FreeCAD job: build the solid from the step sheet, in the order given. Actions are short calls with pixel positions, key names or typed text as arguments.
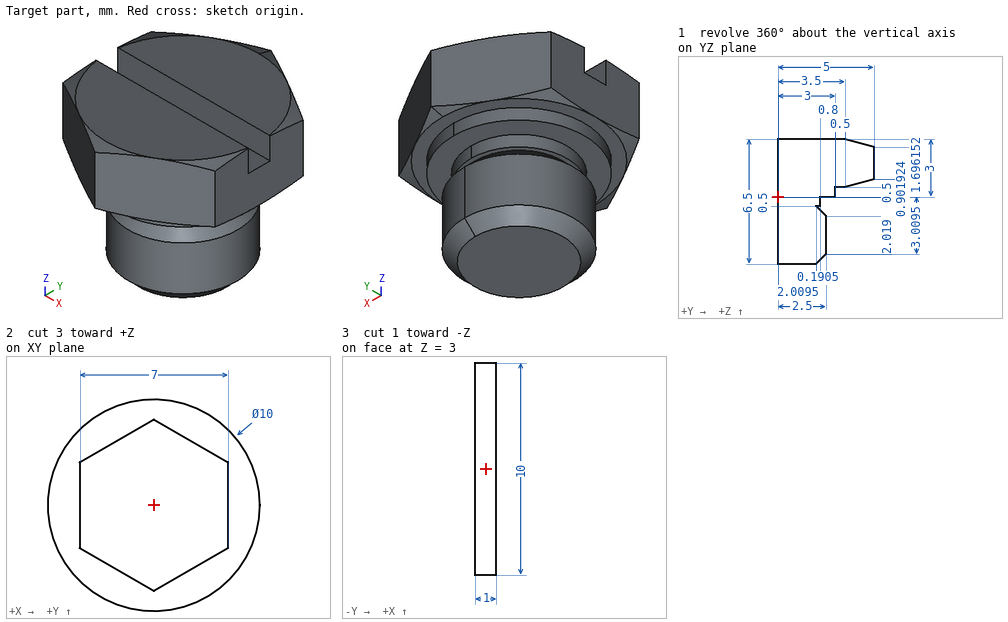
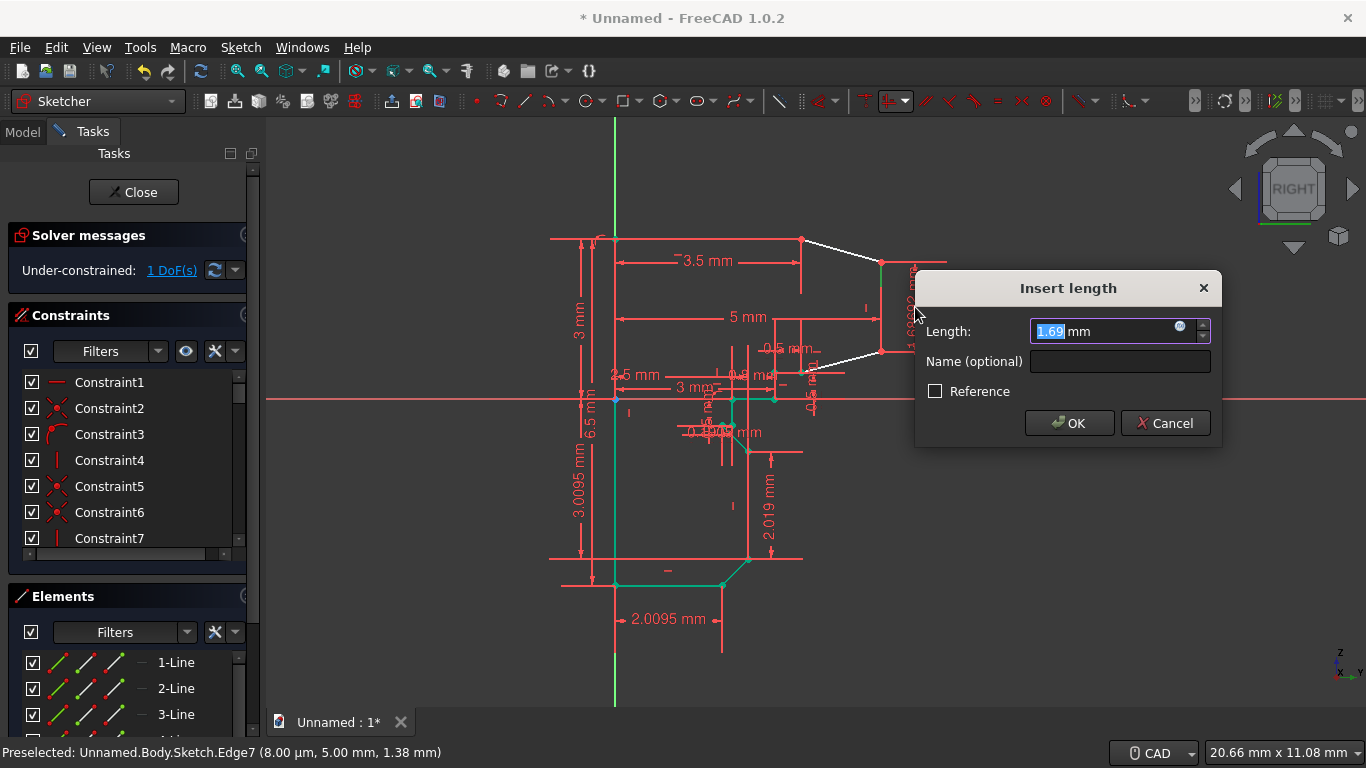
text(1.696152)
key(Return)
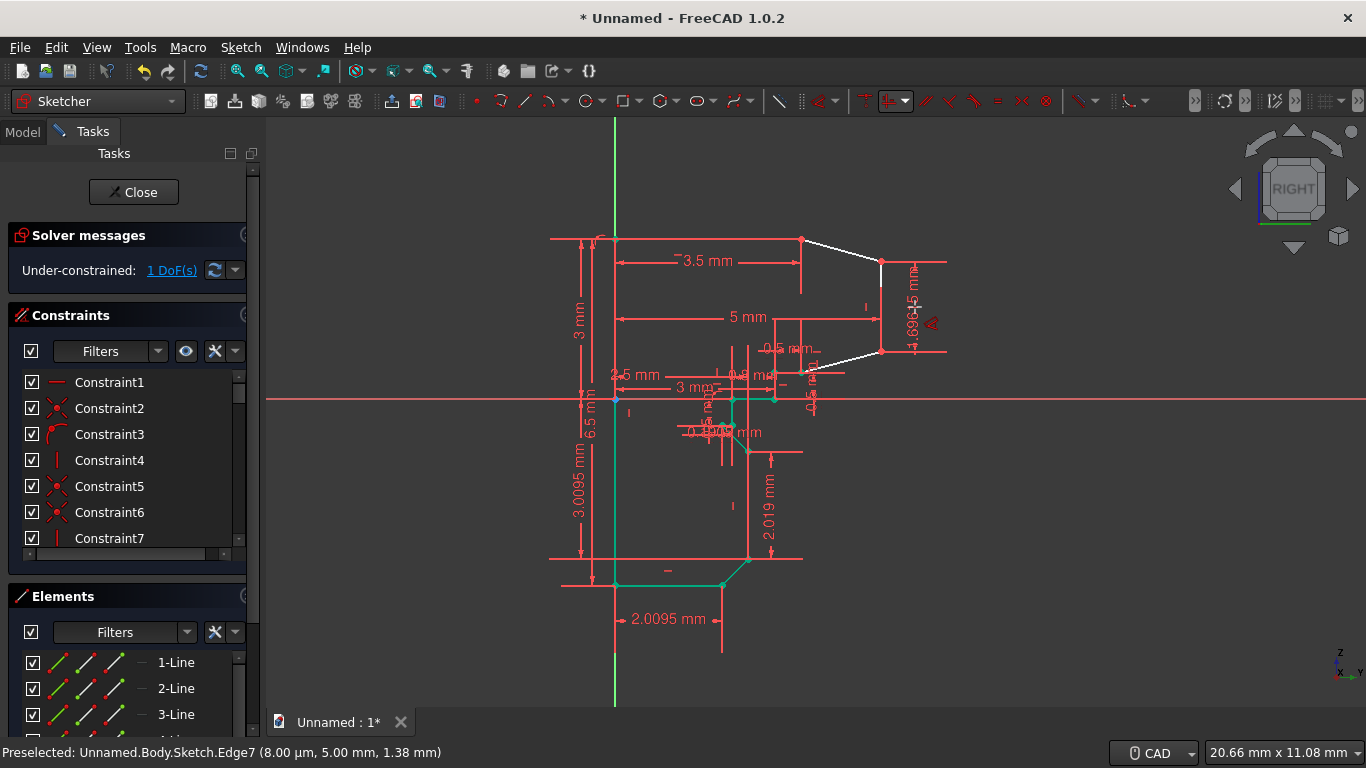
click(881, 352)
click(915, 376)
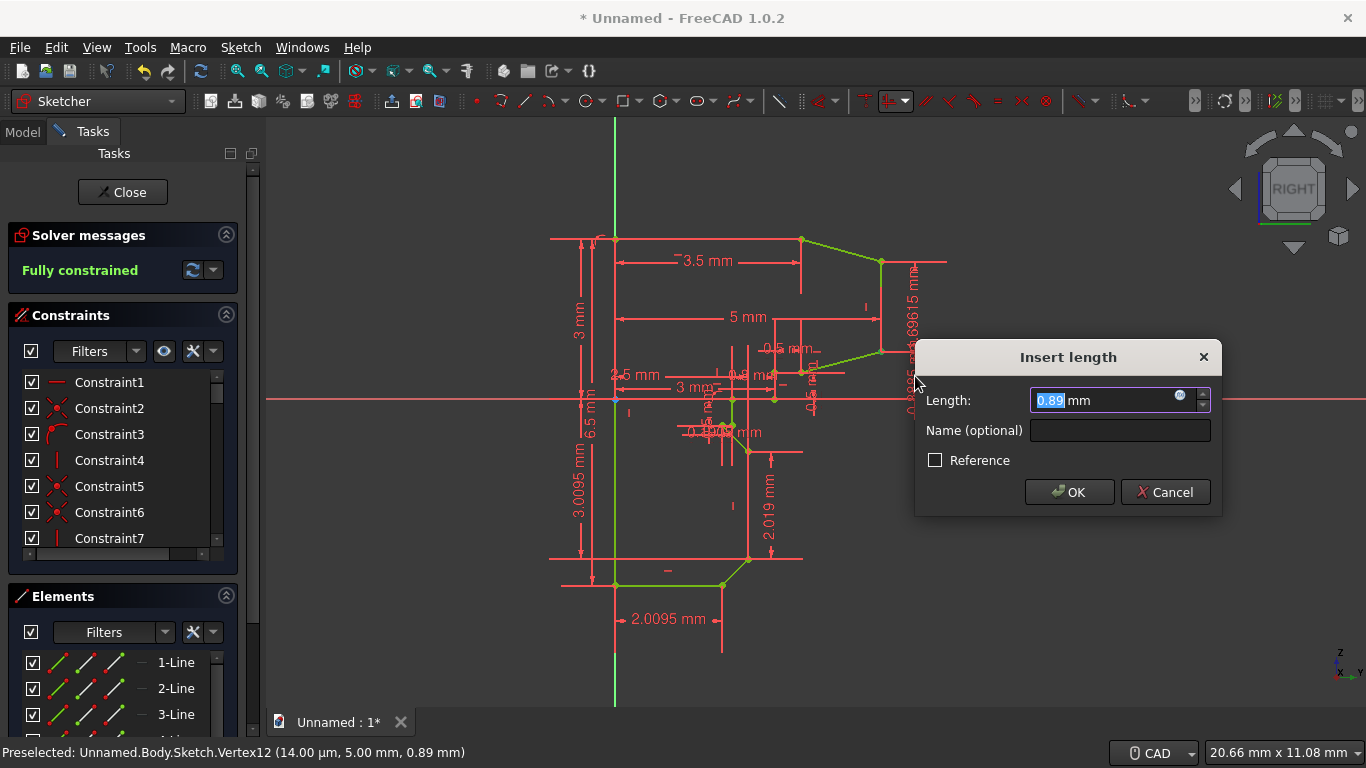
text(0.901924)
key(Return)
key(Escape)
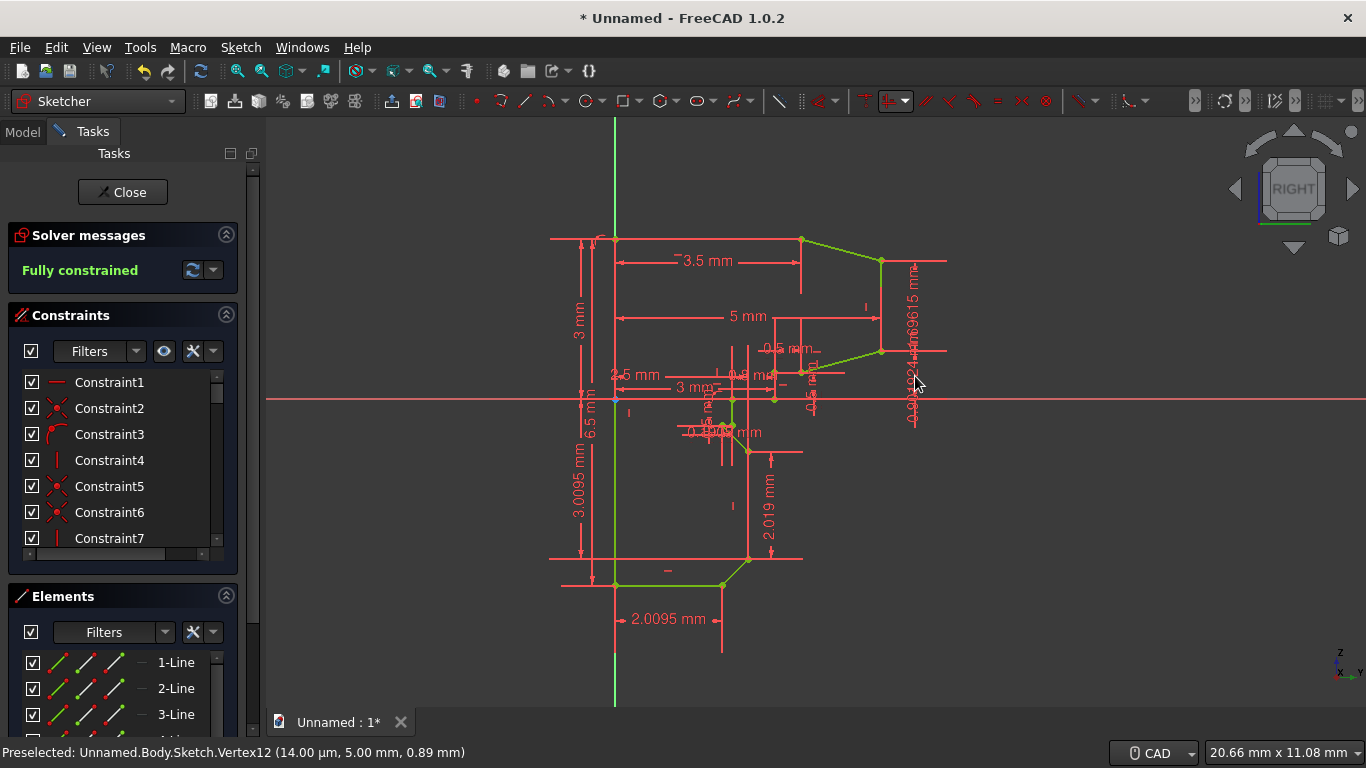
click(123, 192)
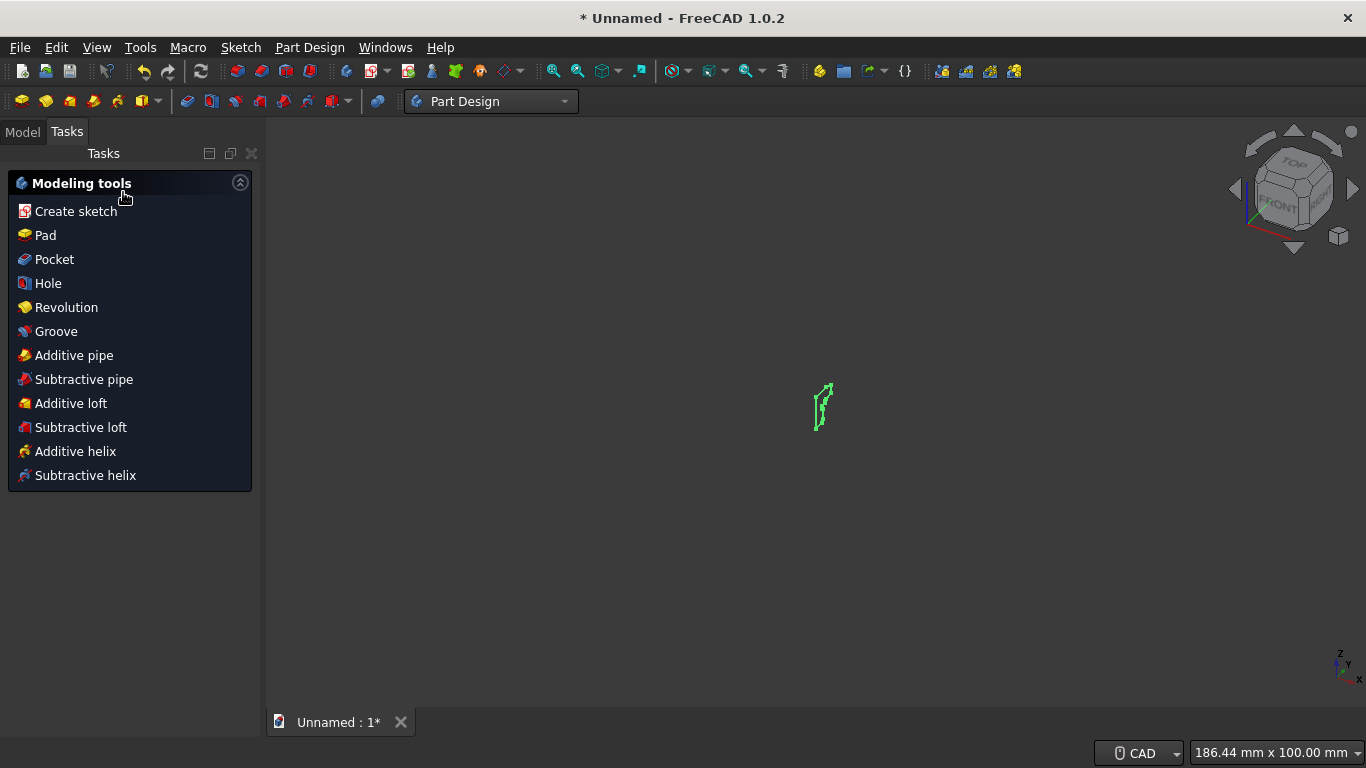
click(46, 102)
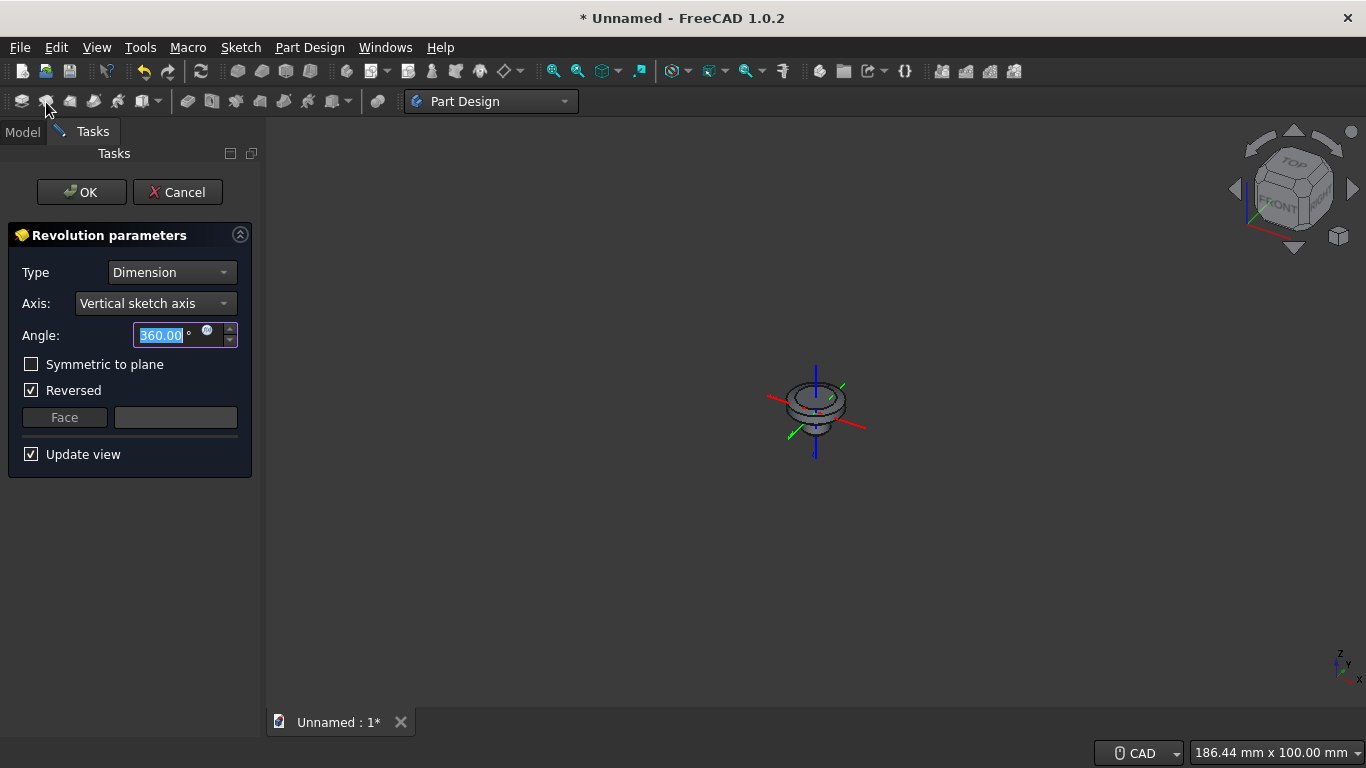
click(82, 192)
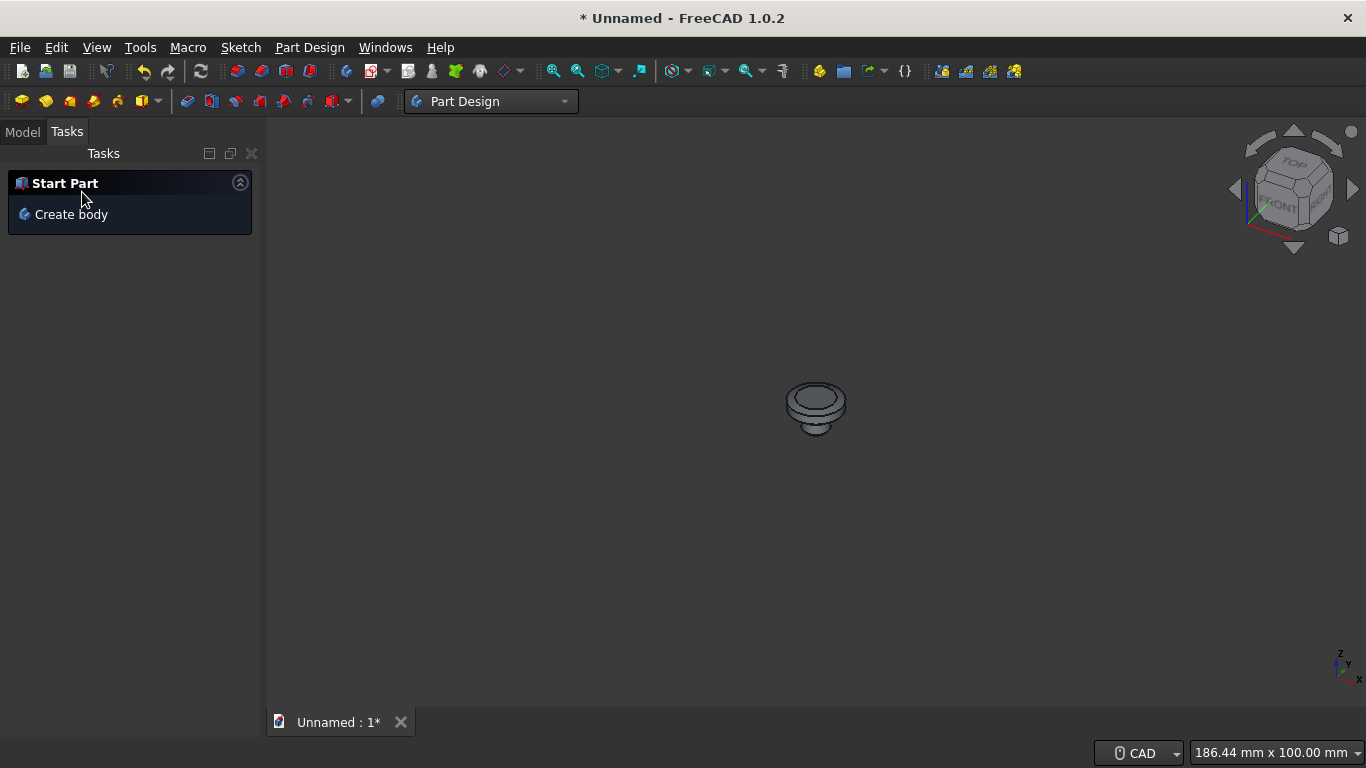
click(554, 72)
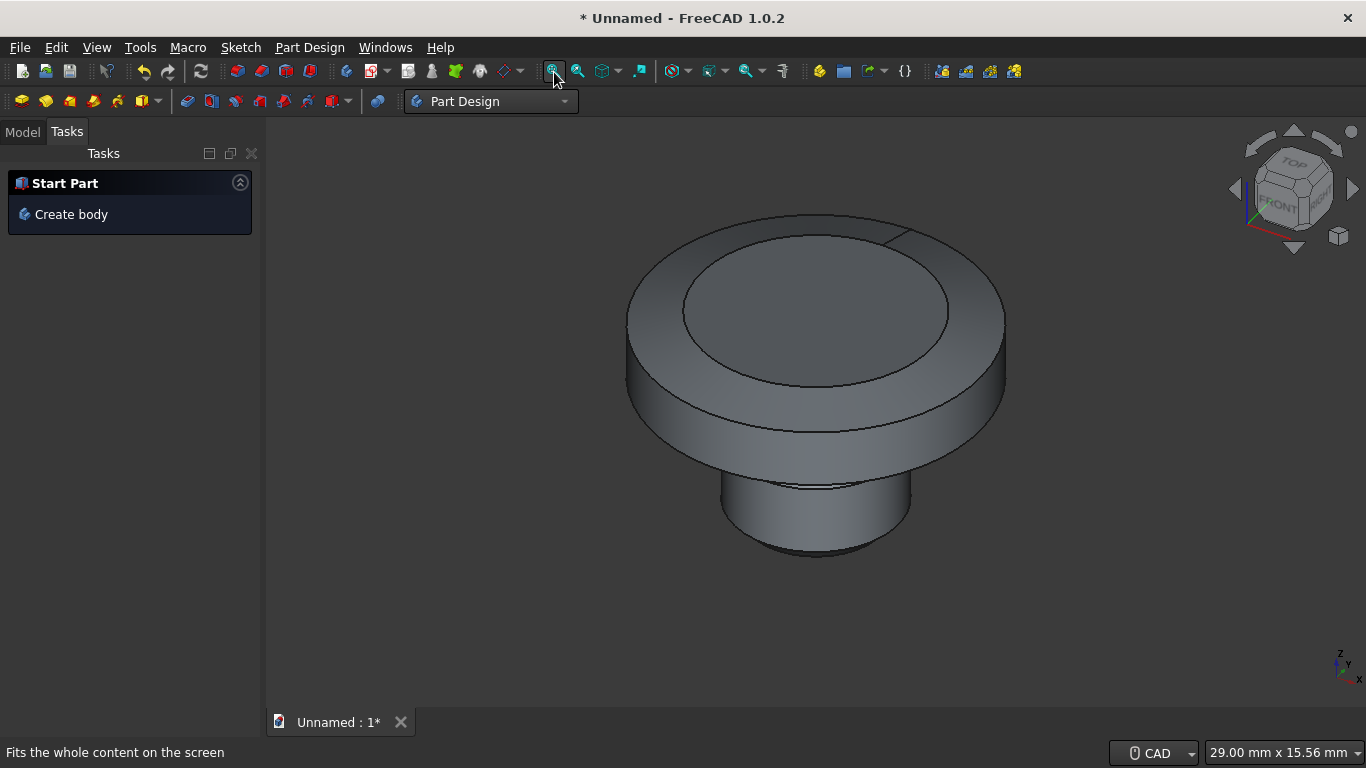
click(372, 72)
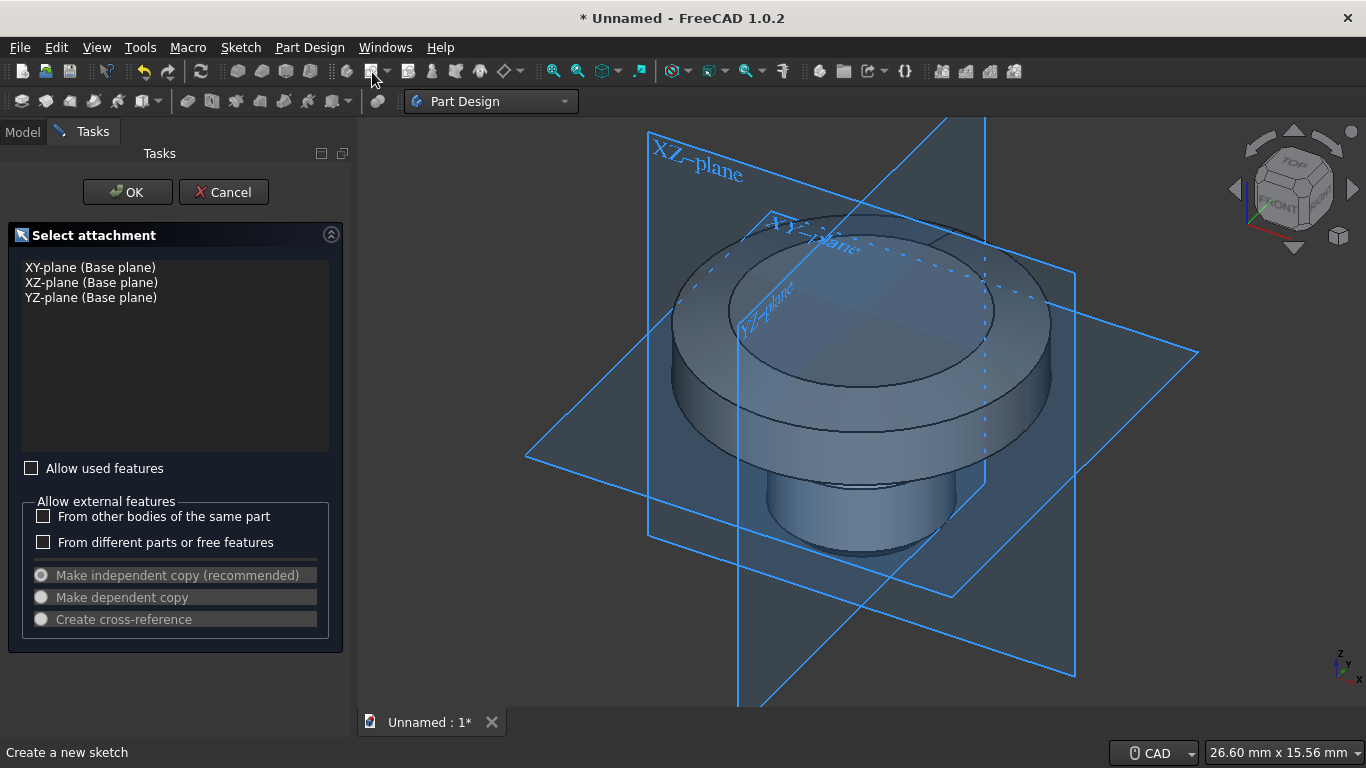
click(82, 268)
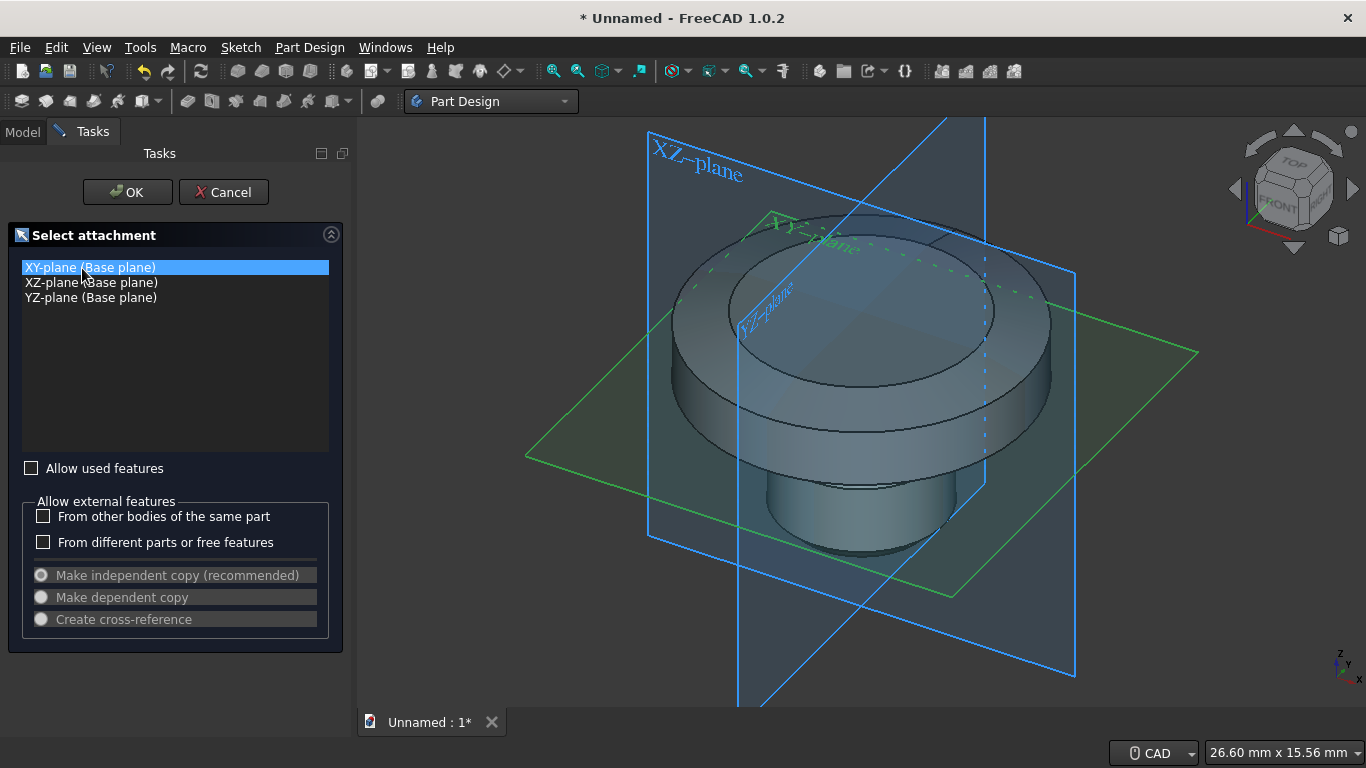
click(128, 192)